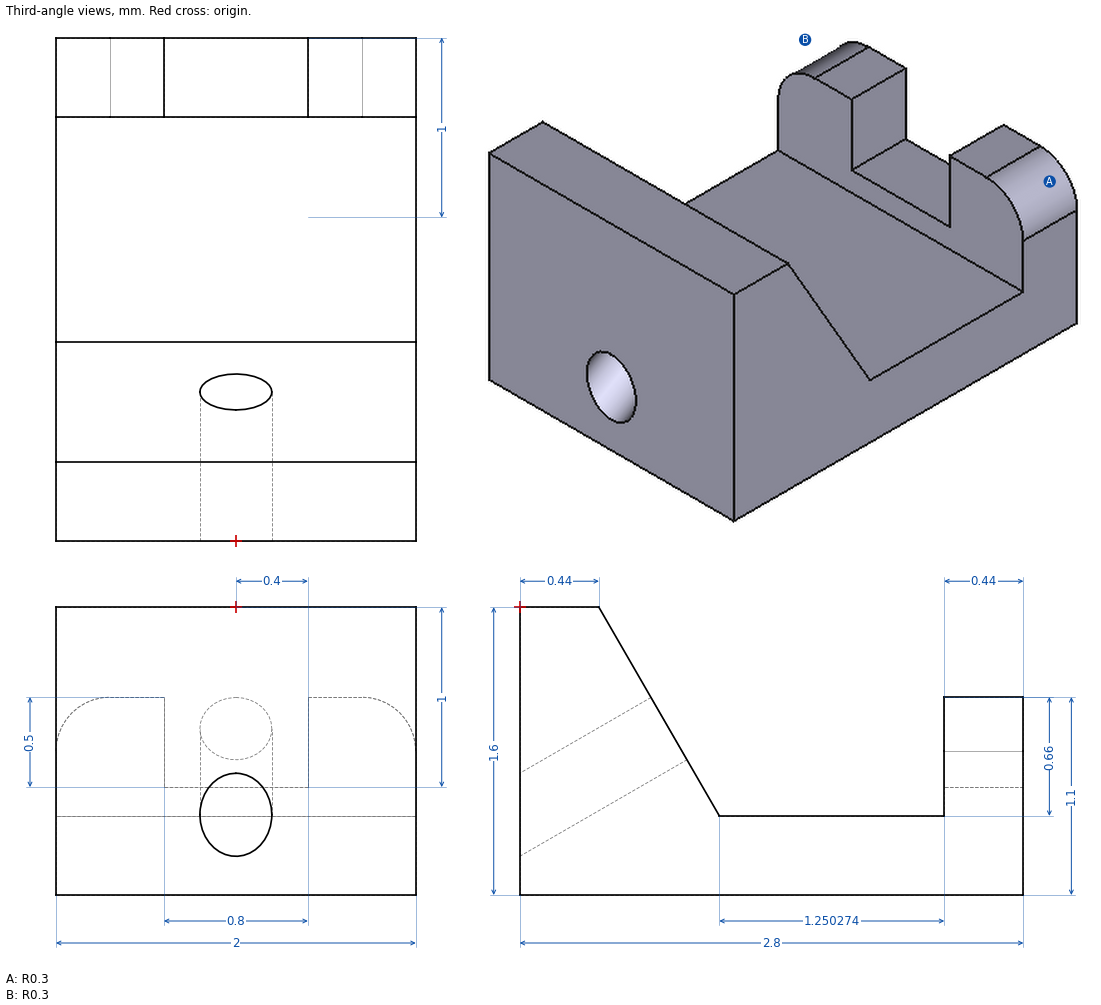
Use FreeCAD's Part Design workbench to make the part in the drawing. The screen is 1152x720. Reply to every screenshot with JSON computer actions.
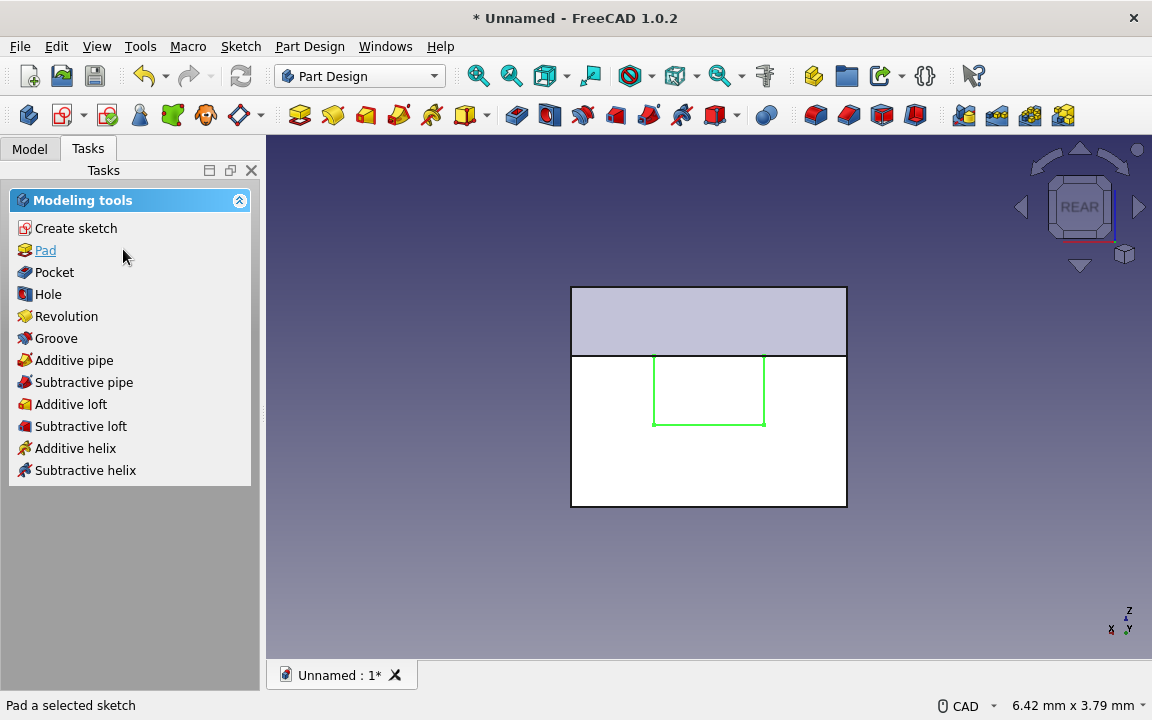
{"action": "left_click", "coordinate": [517, 116]}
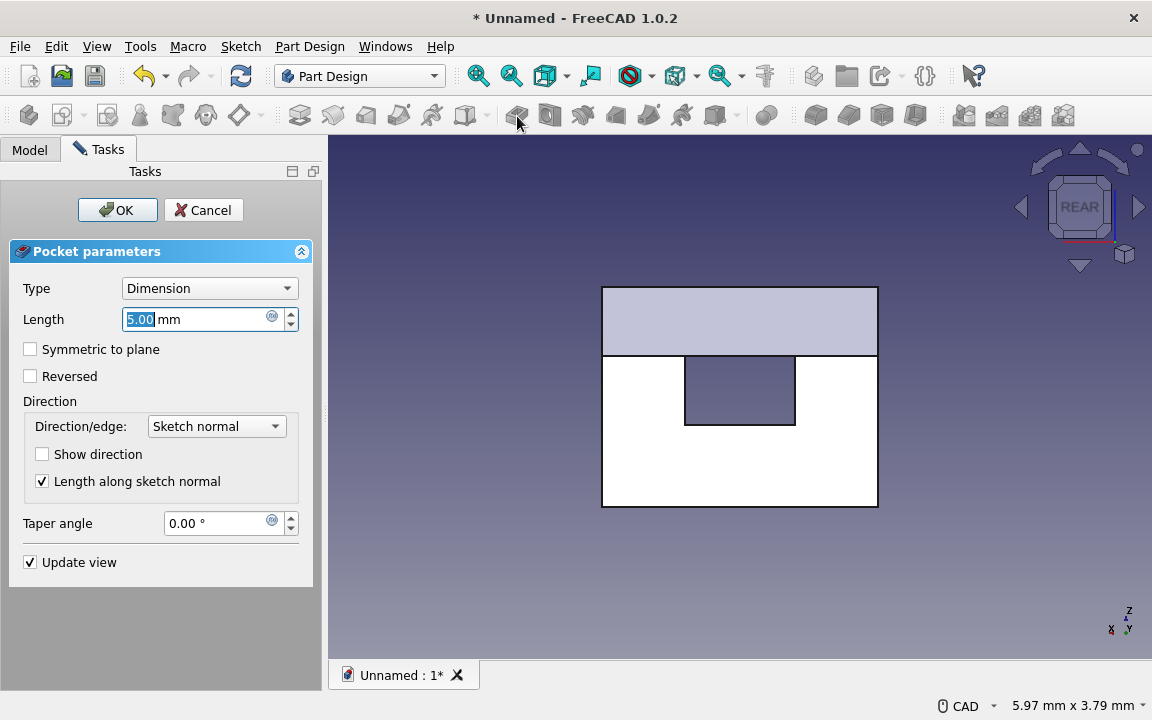
{"action": "type", "text": "1"}
{"action": "key", "text": "Tab"}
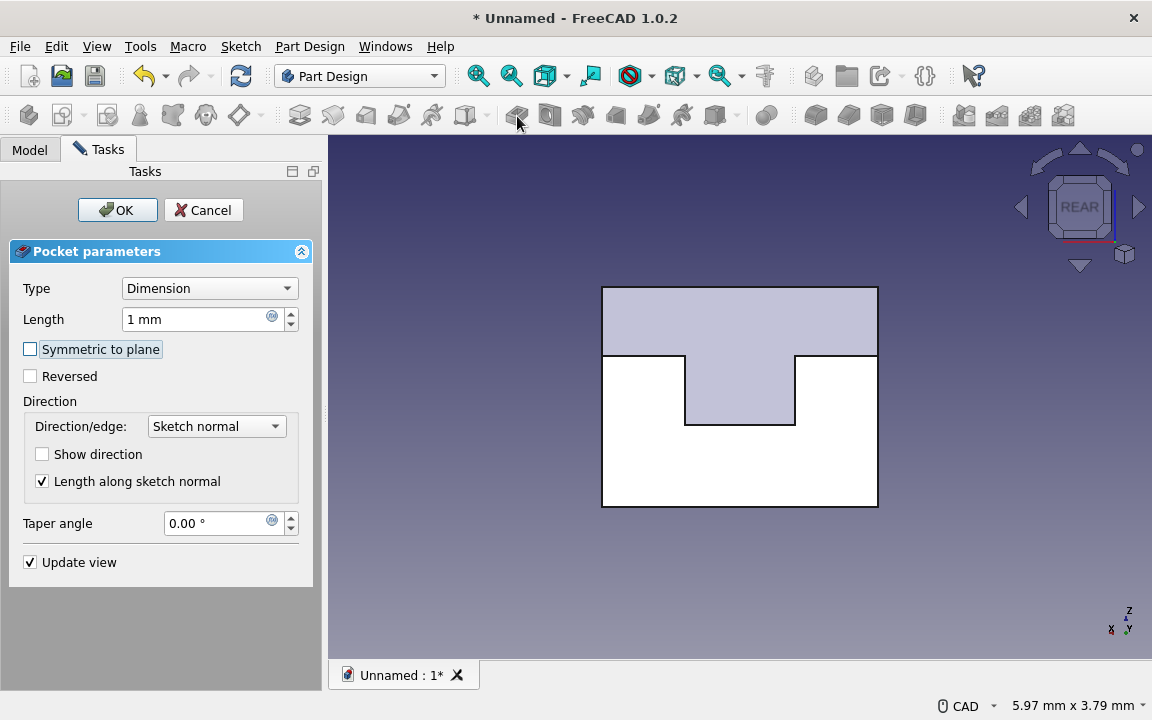
{"action": "left_click", "coordinate": [118, 210]}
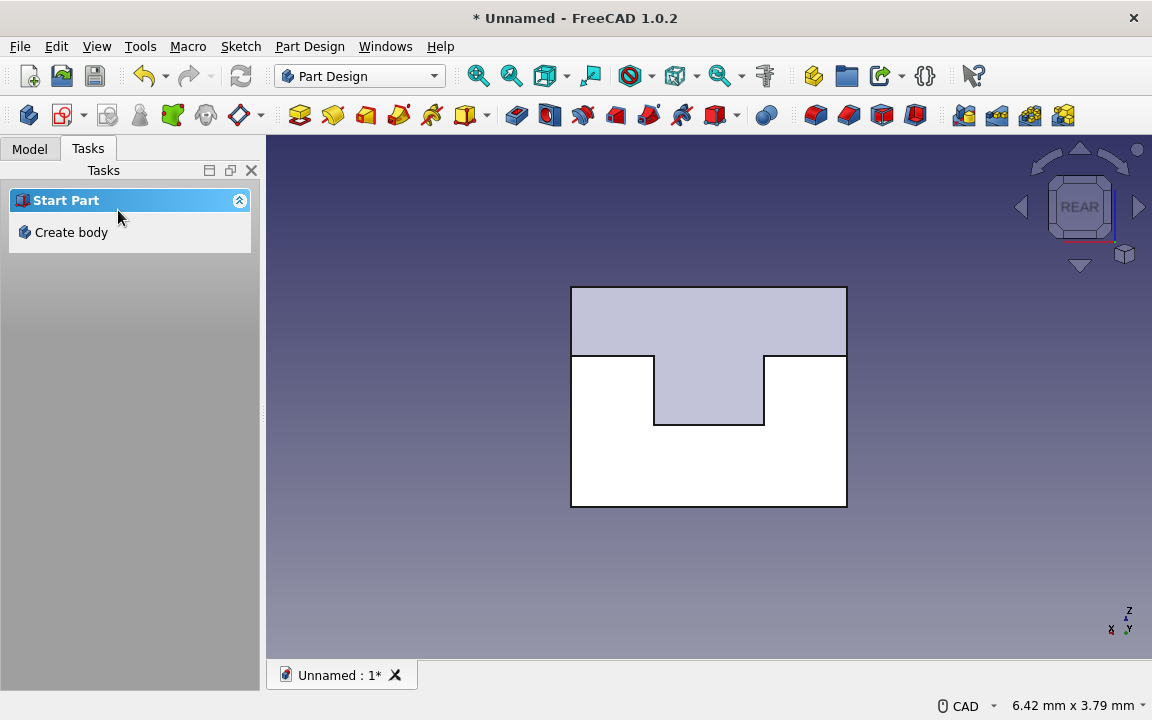
{"action": "key", "text": "v f"}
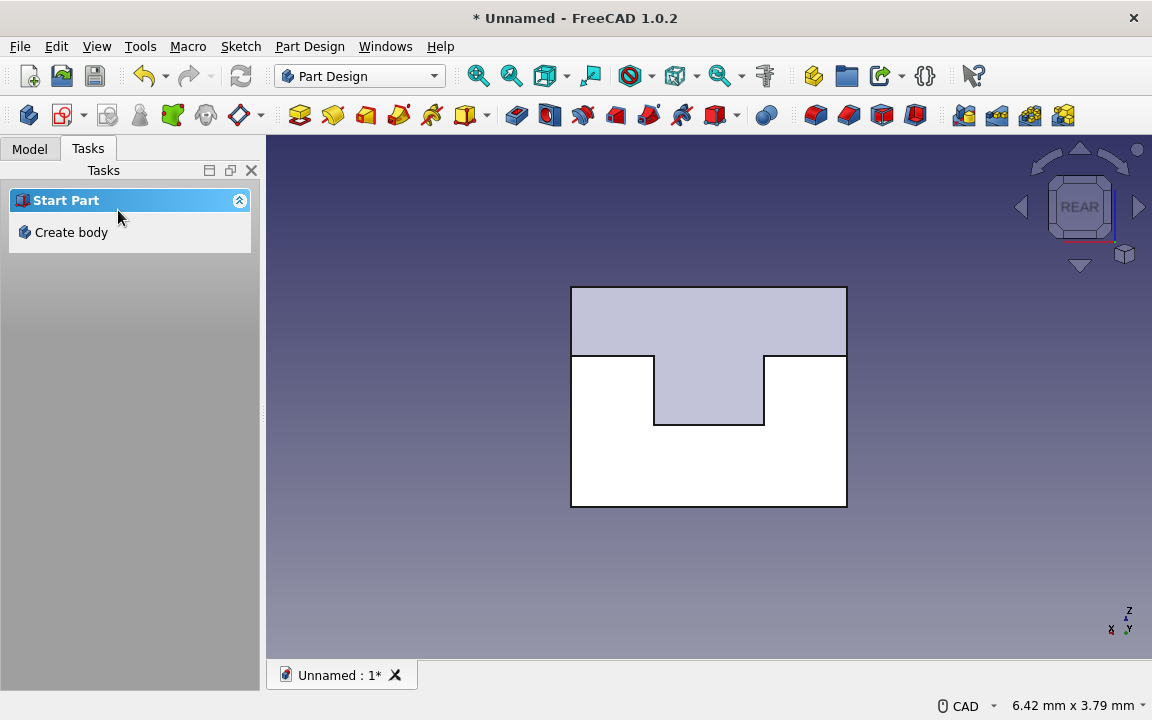
{"action": "key", "text": "0"}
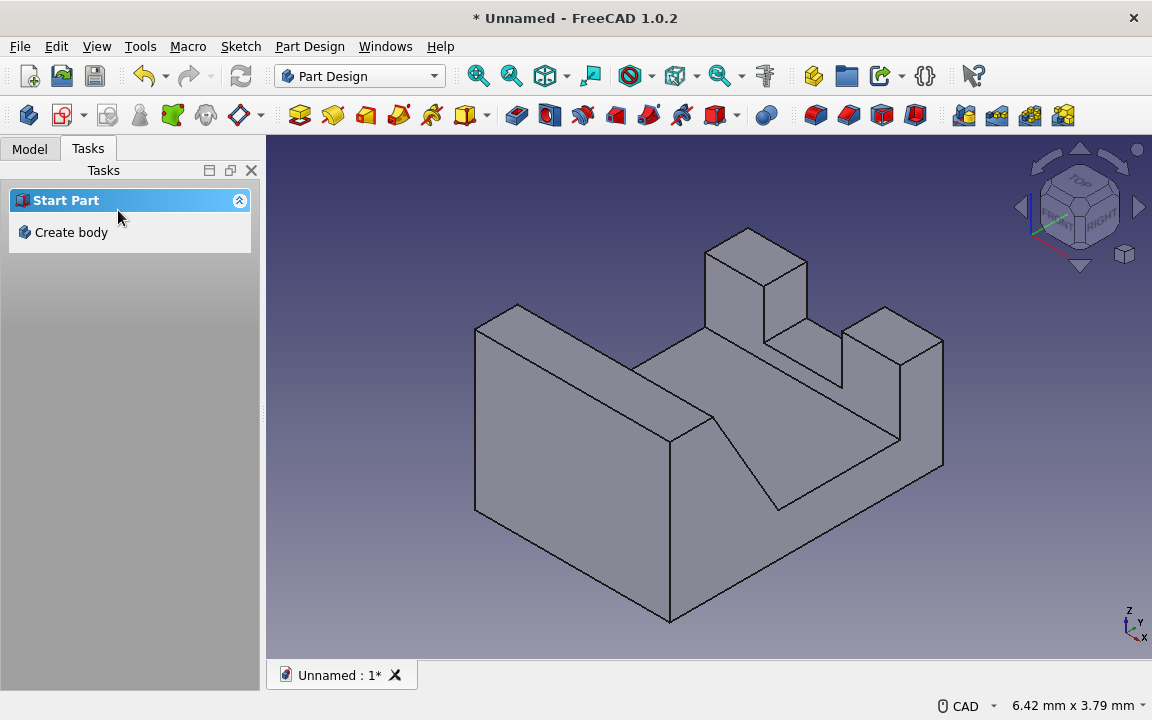
{"action": "left_click", "coordinate": [922, 352]}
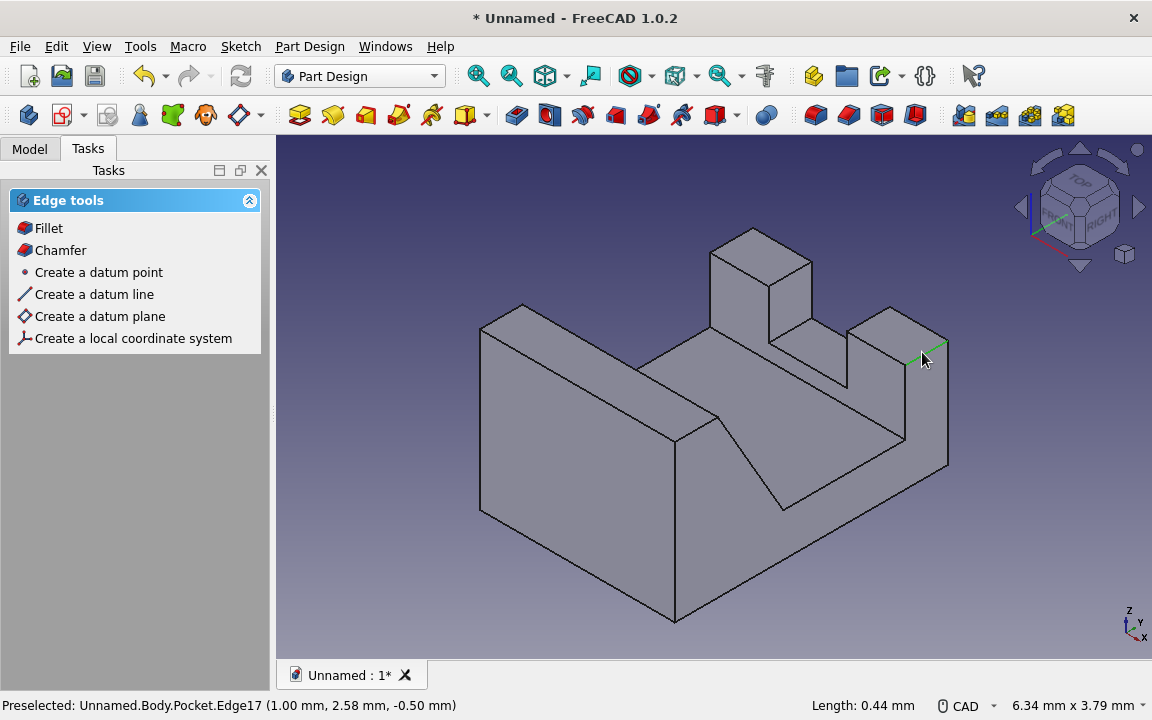
{"action": "left_click", "coordinate": [816, 116]}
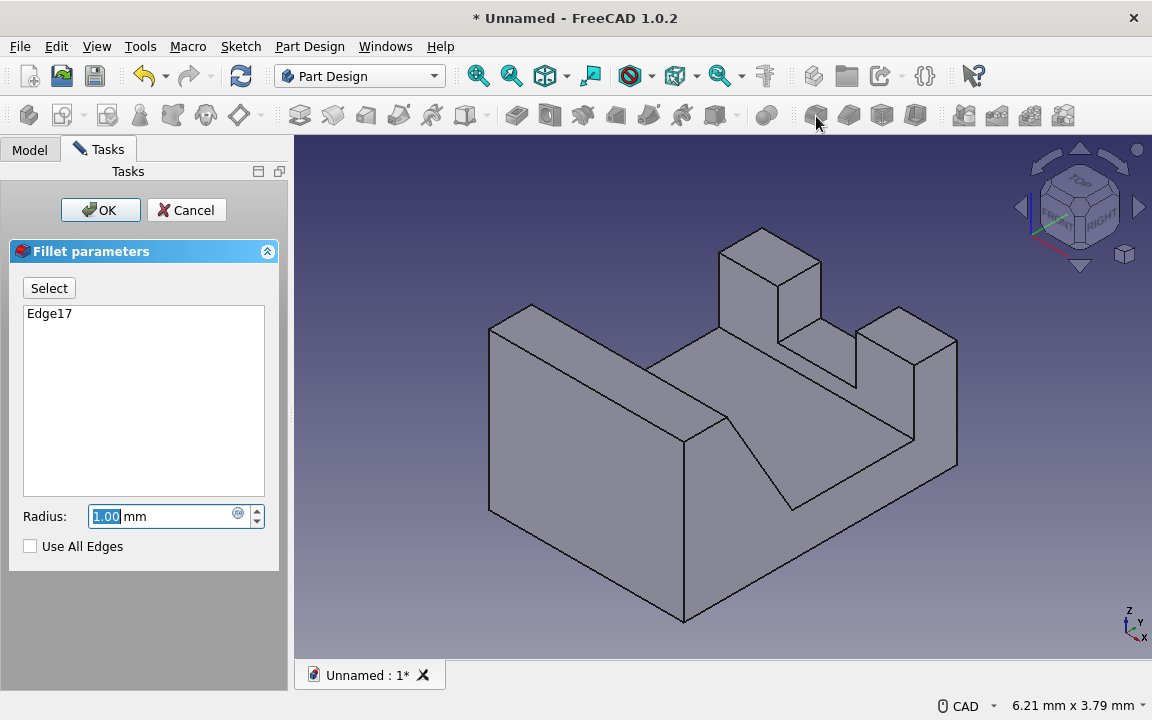
{"action": "type", "text": "0.3"}
{"action": "key", "text": "Tab"}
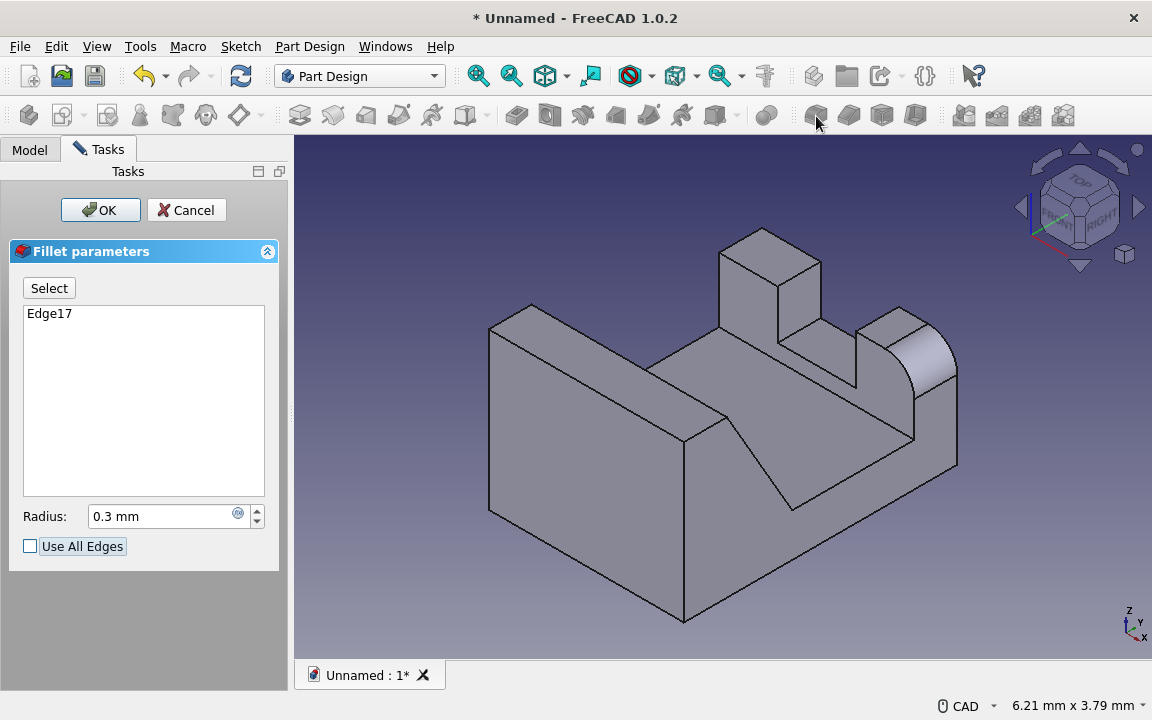
{"action": "left_click", "coordinate": [101, 210]}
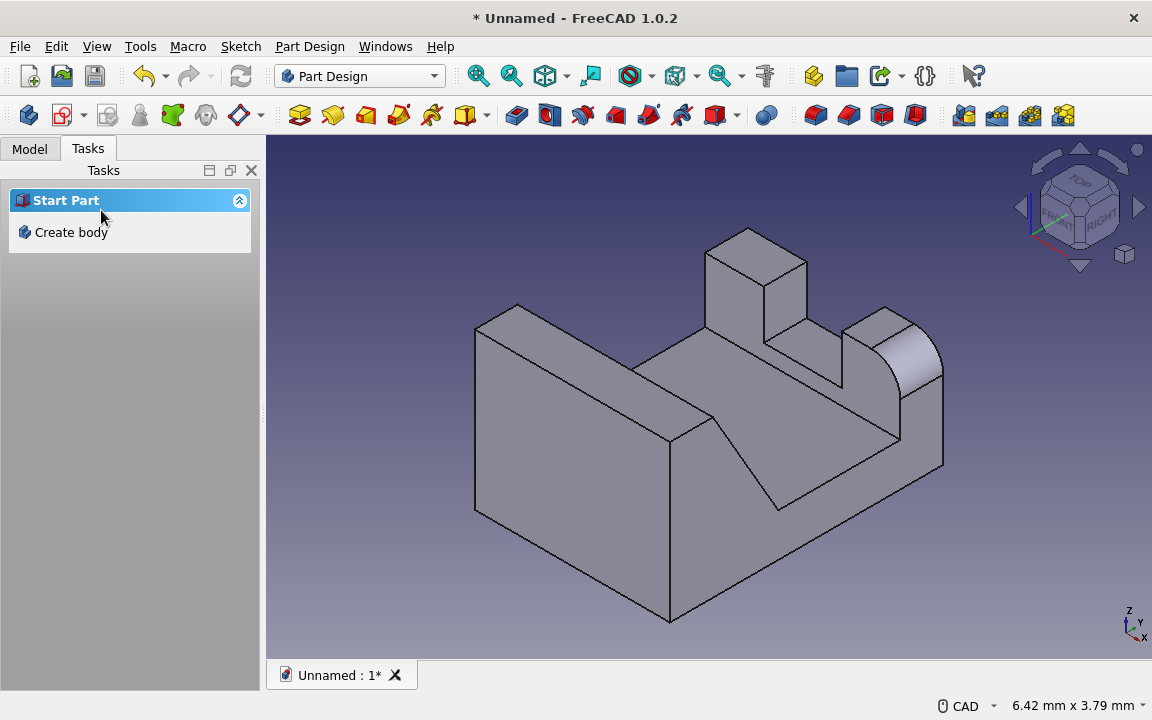
{"action": "key", "text": "2"}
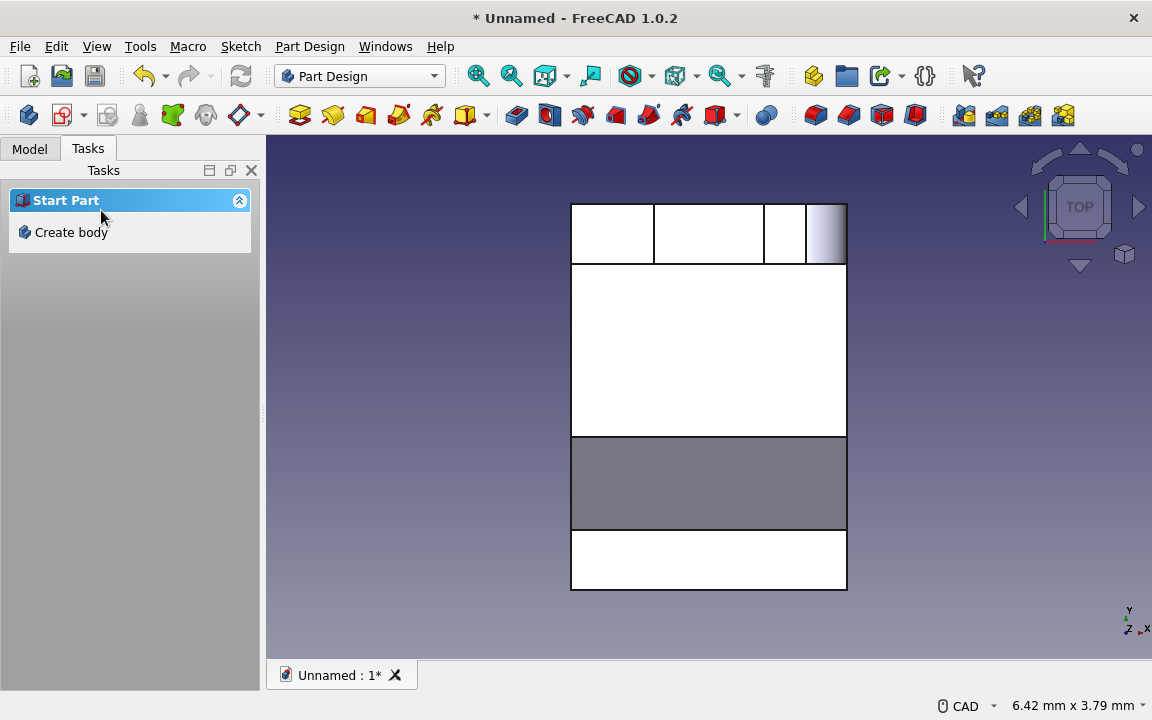
{"action": "left_click", "coordinate": [571, 233]}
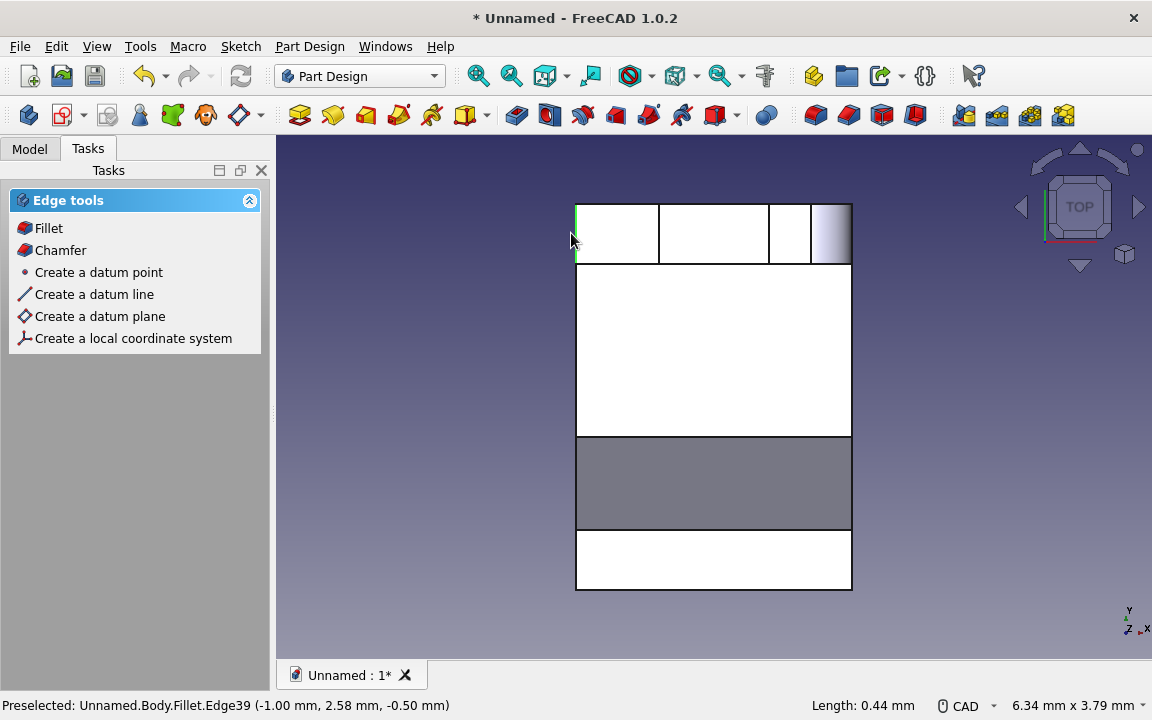
{"action": "left_click", "coordinate": [816, 116]}